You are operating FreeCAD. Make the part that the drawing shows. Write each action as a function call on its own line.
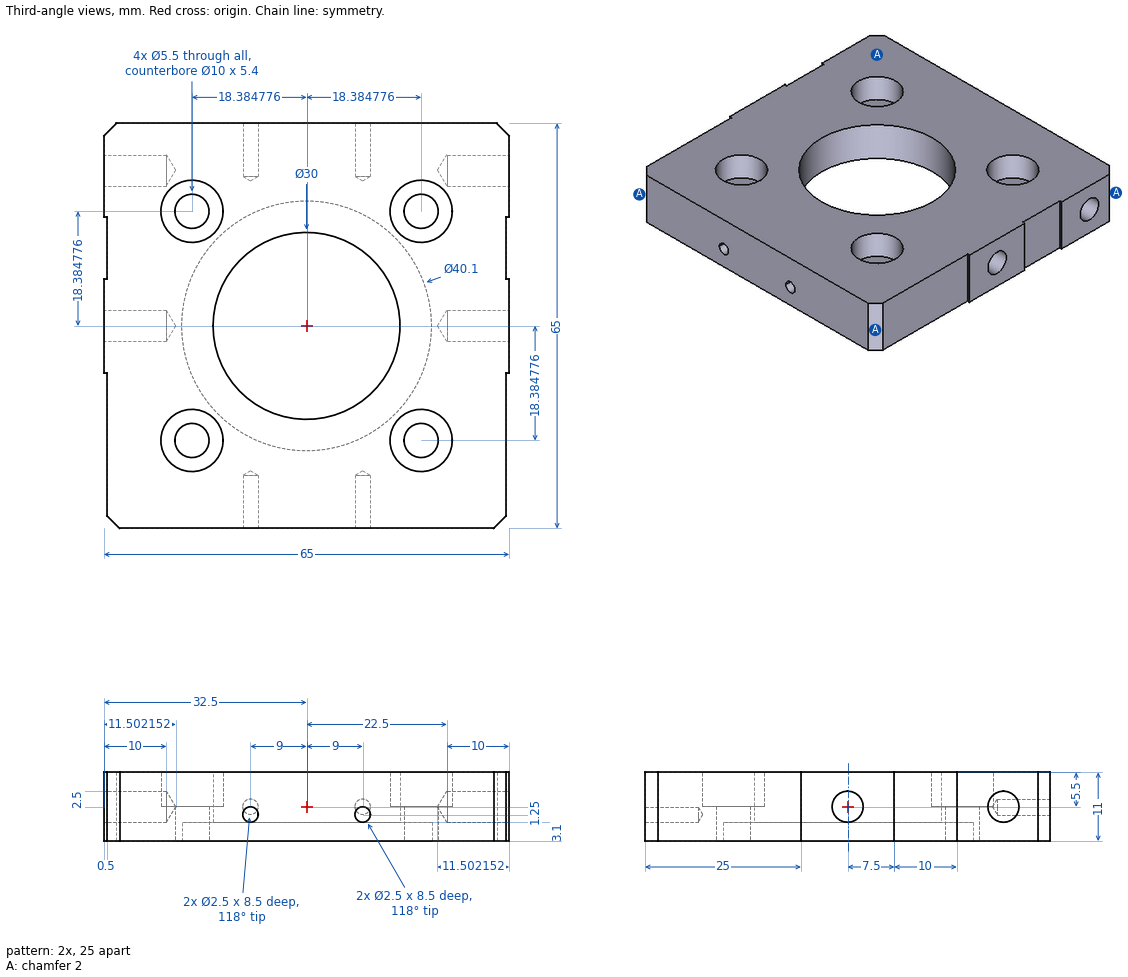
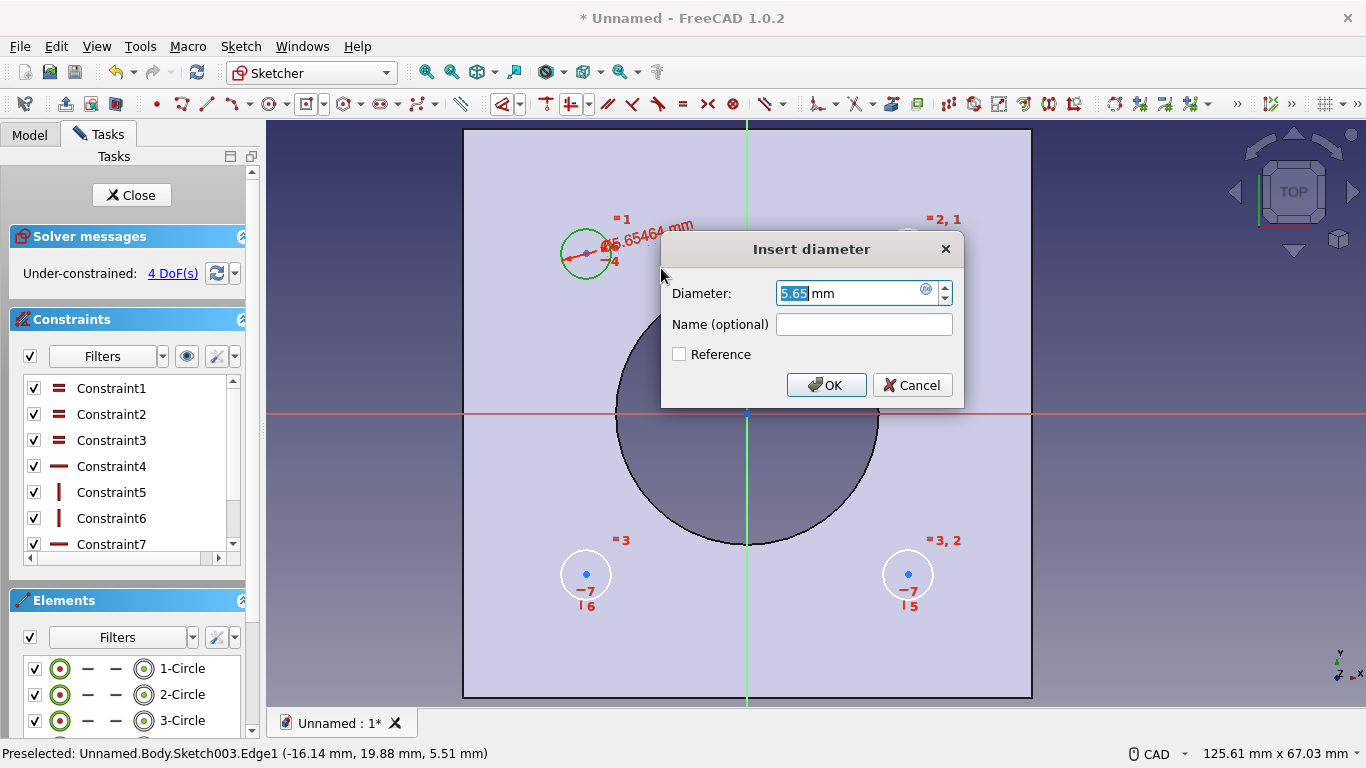
text(5.5)
key(Return)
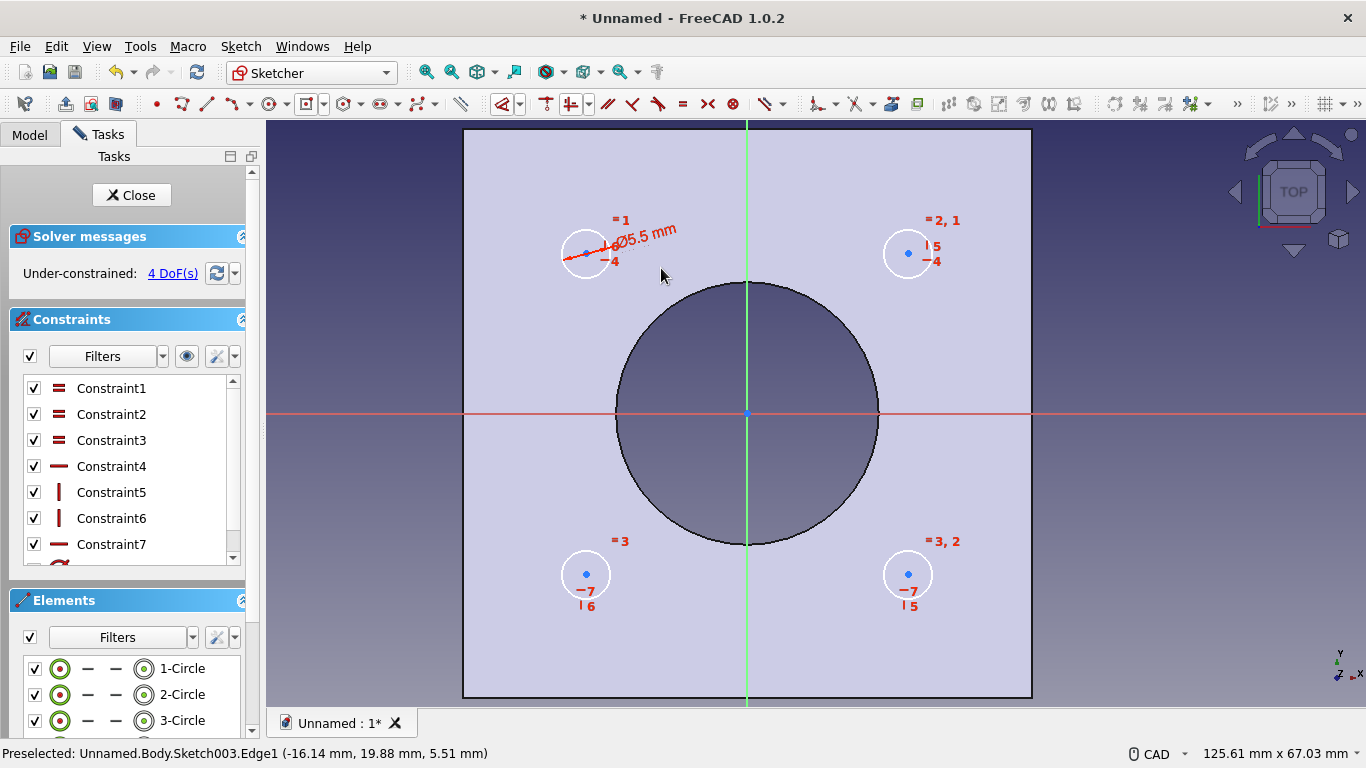
click(586, 254)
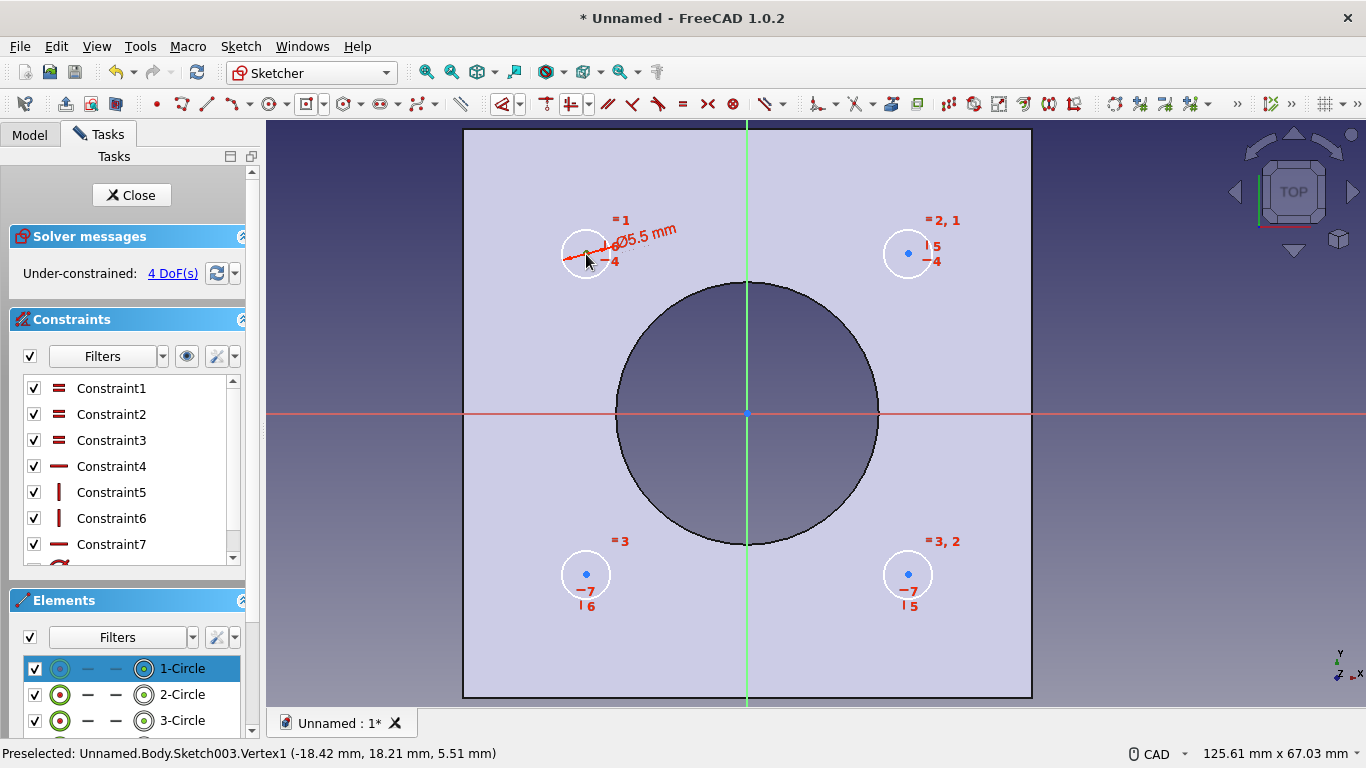
click(520, 104)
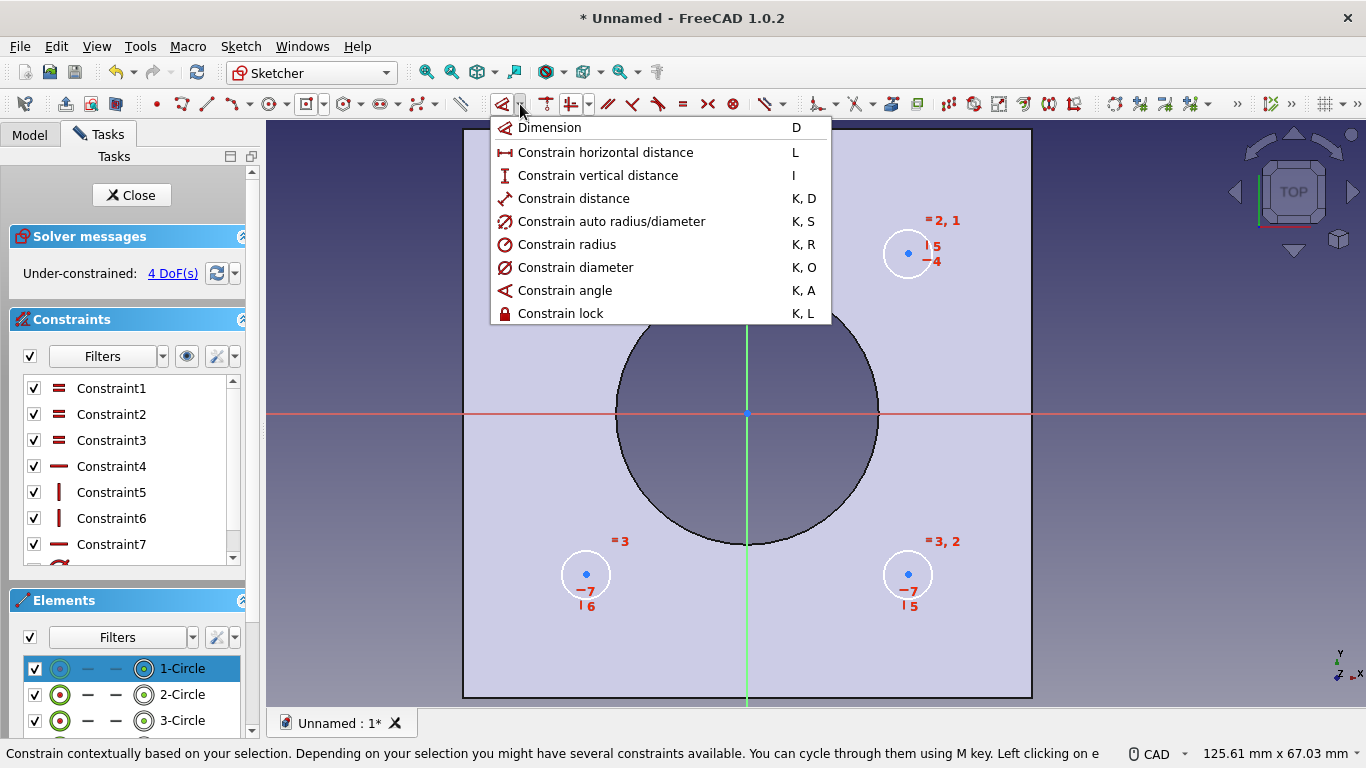
click(661, 152)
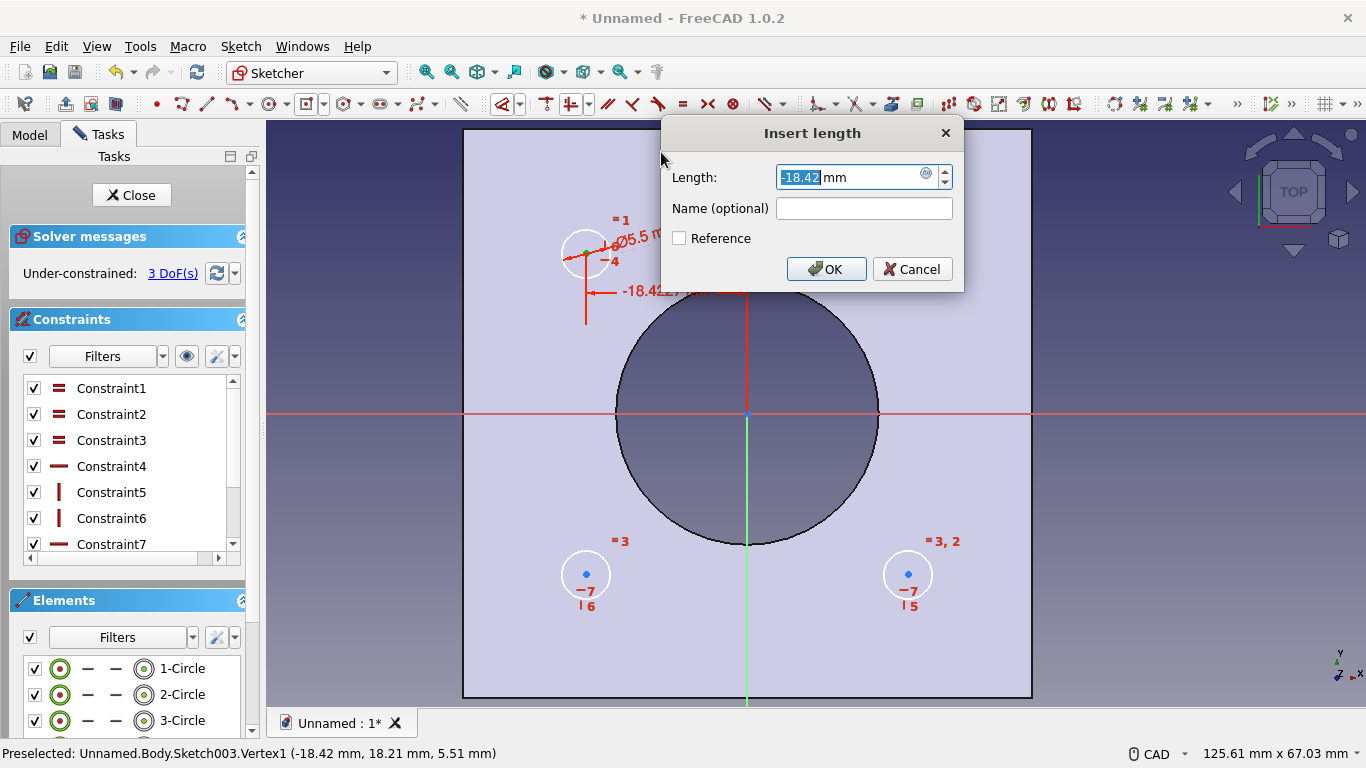
text(-18.384776)
key(Return)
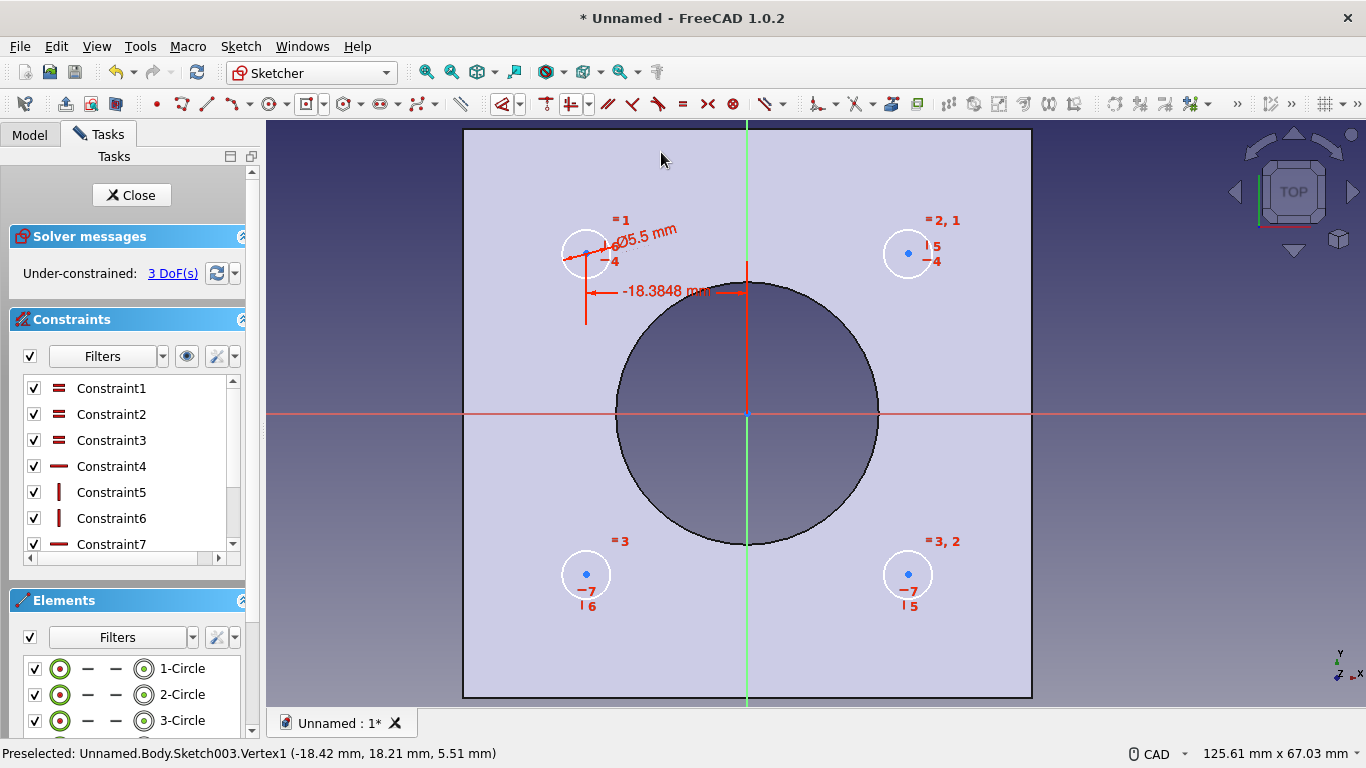
click(586, 254)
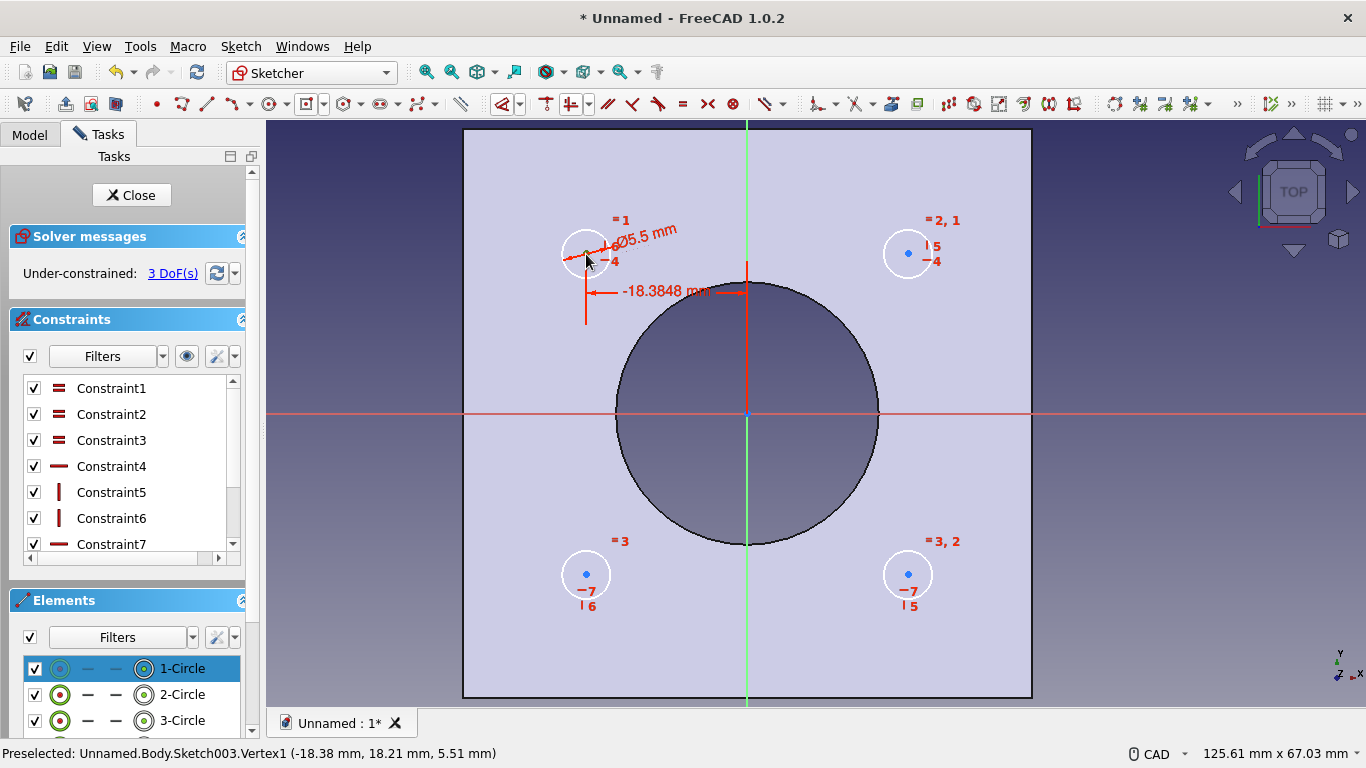
click(520, 104)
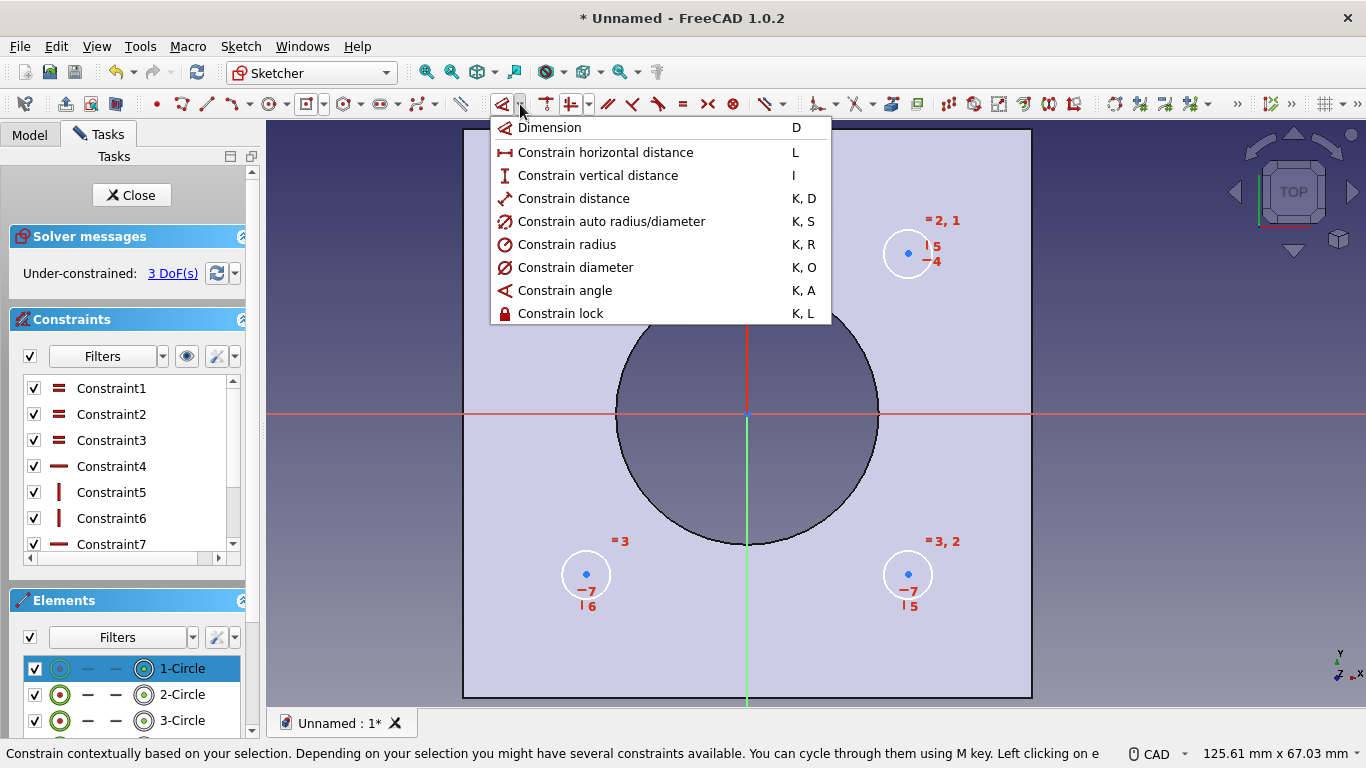
click(661, 176)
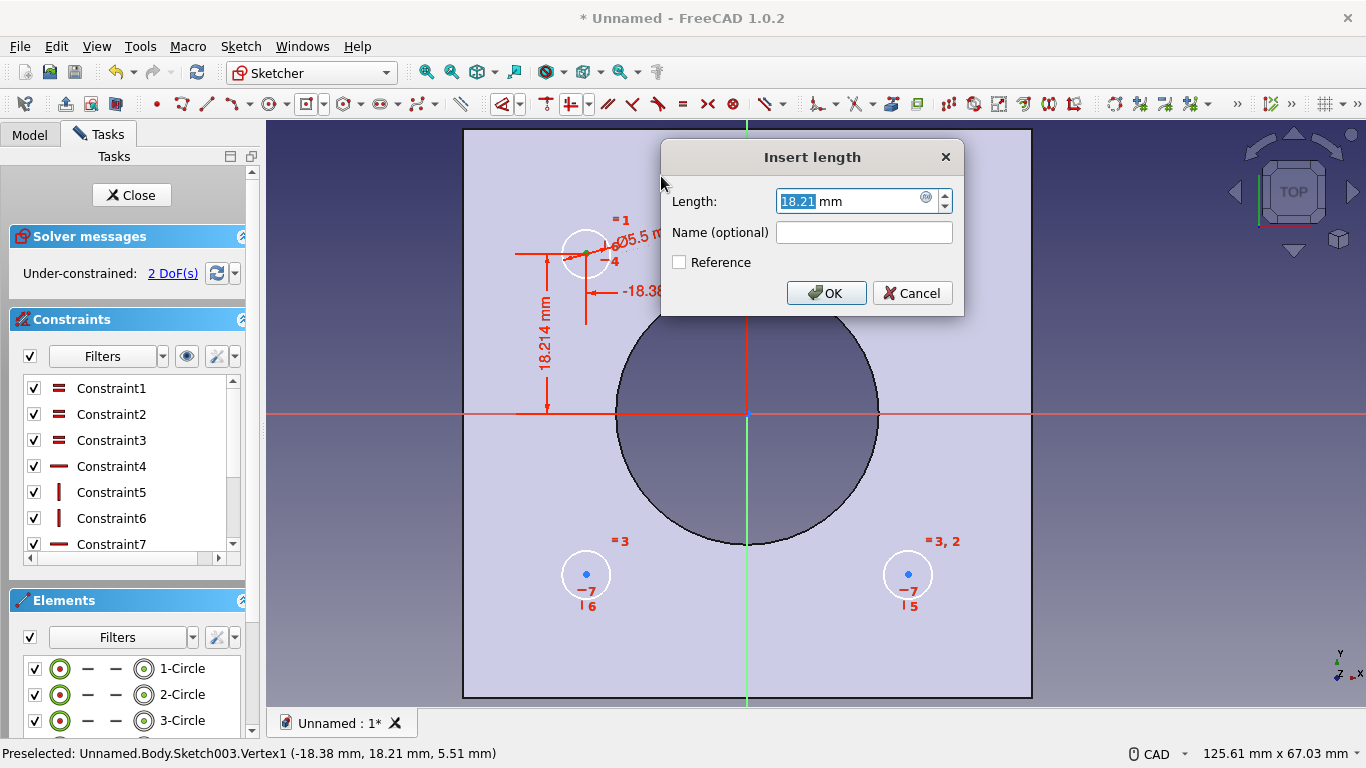
text(18.384776)
key(Return)